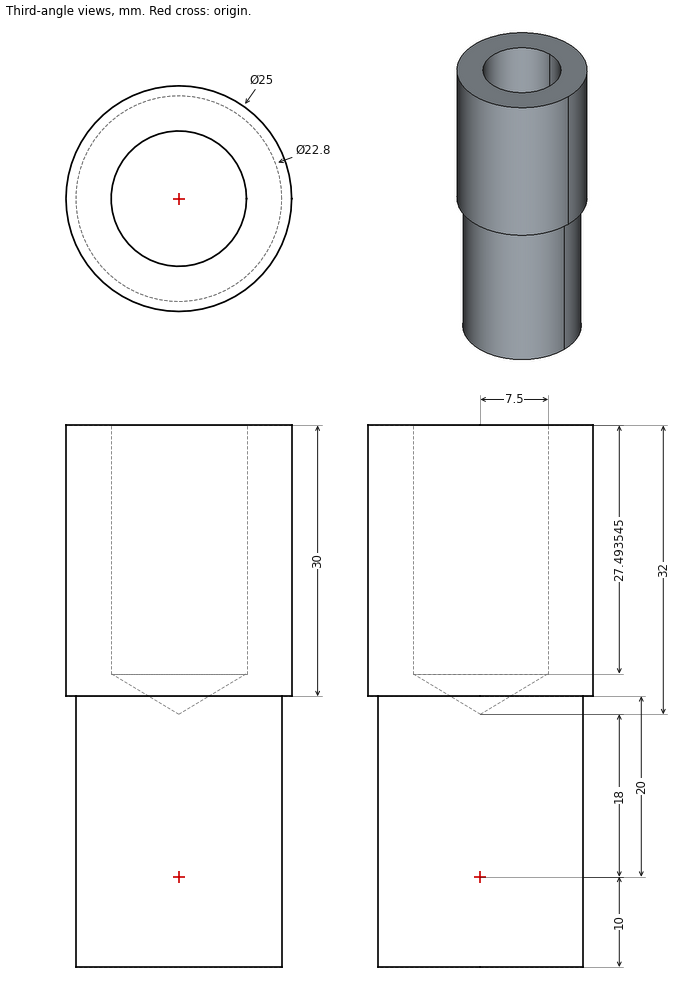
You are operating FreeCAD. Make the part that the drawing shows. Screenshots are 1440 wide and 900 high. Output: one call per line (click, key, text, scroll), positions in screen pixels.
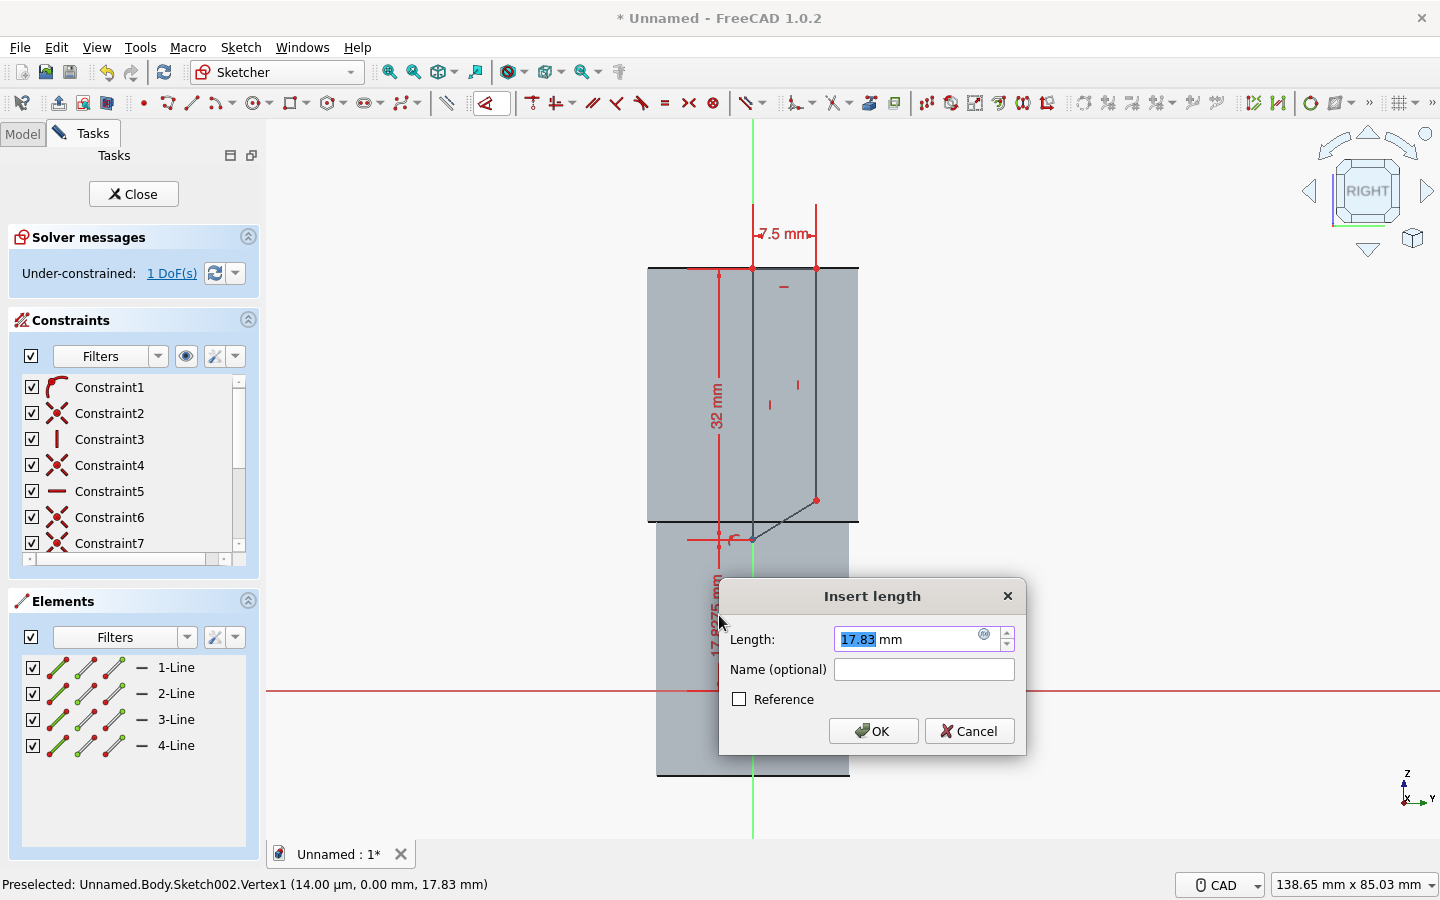
text(18)
key(Return)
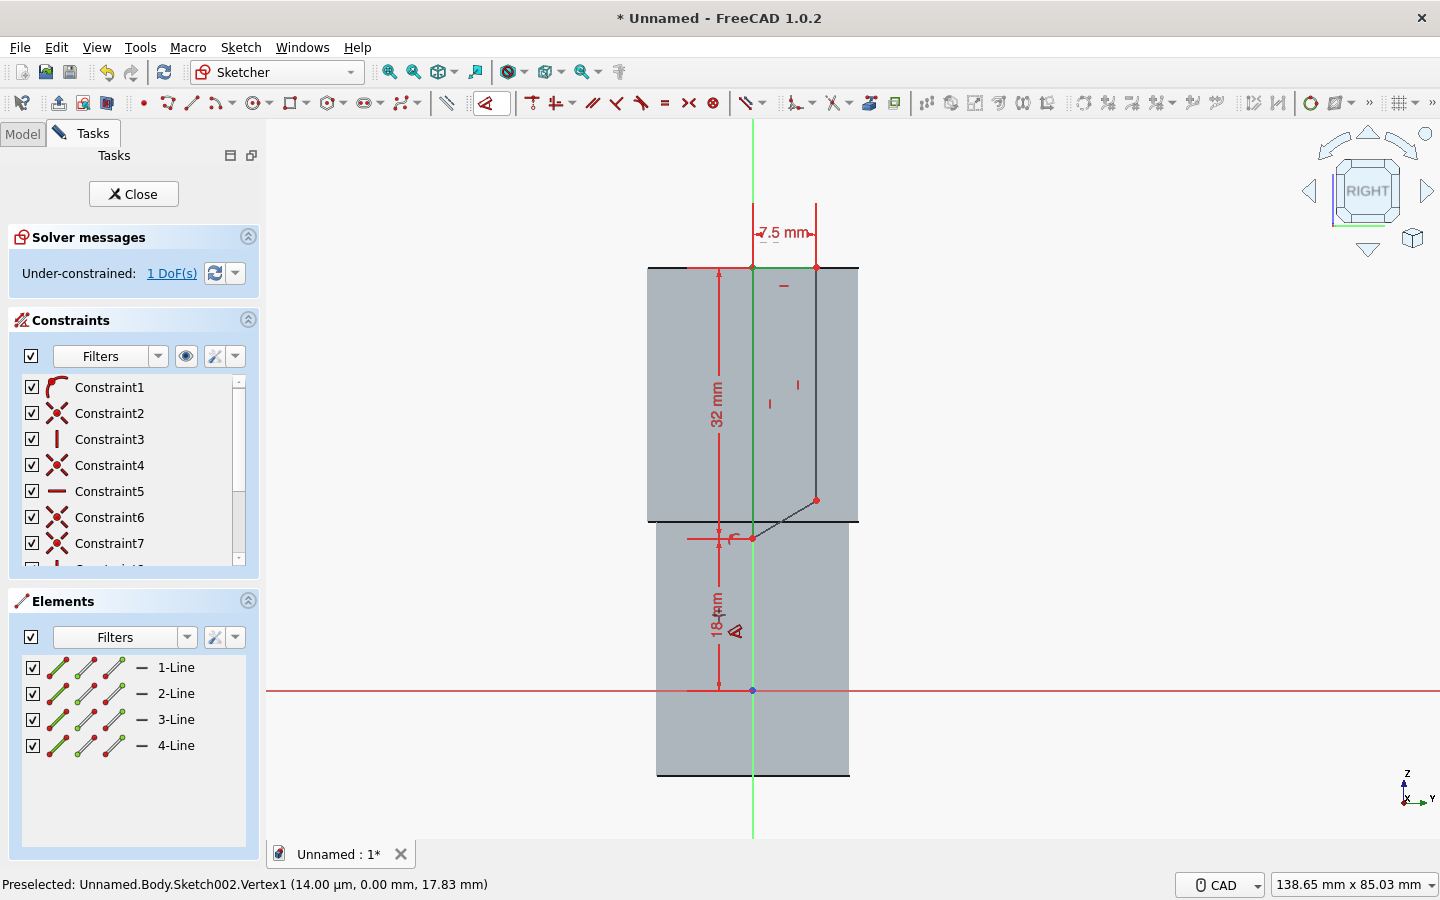
click(816, 431)
click(850, 384)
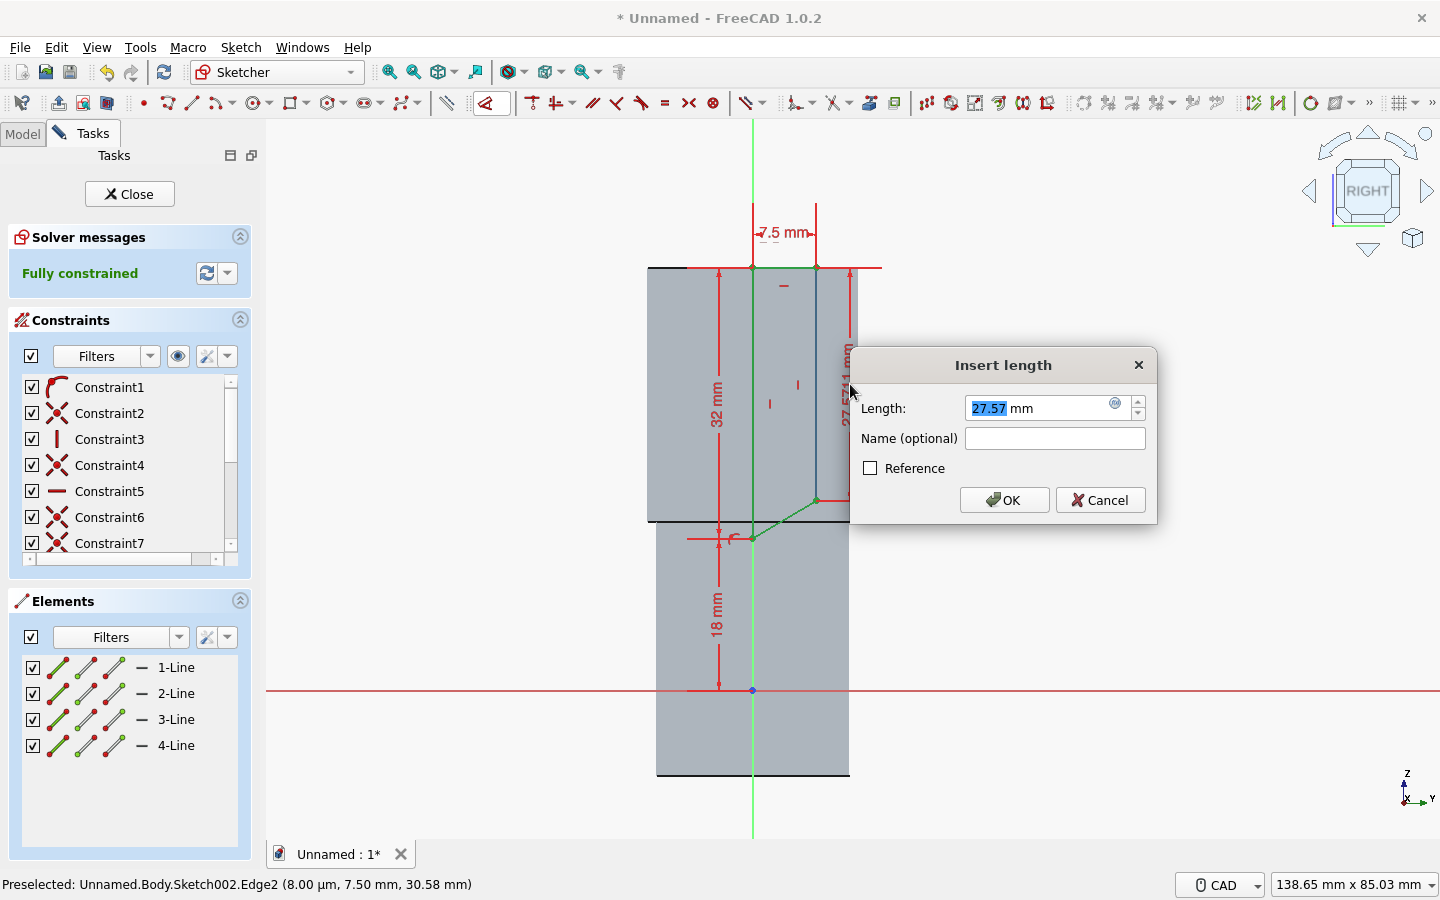
text(27.493545)
key(Return)
key(Escape)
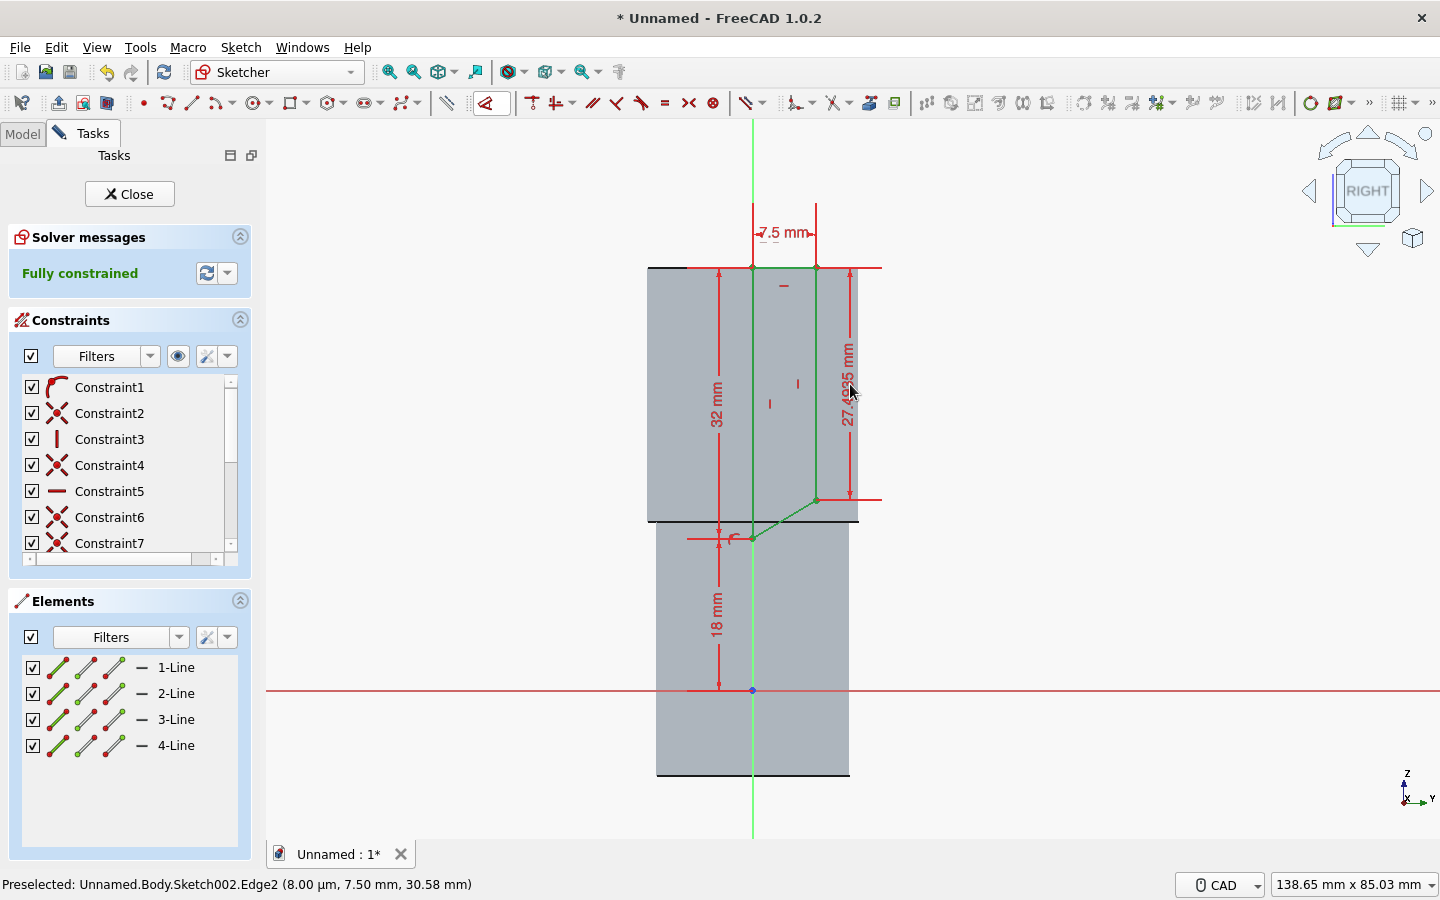
click(130, 194)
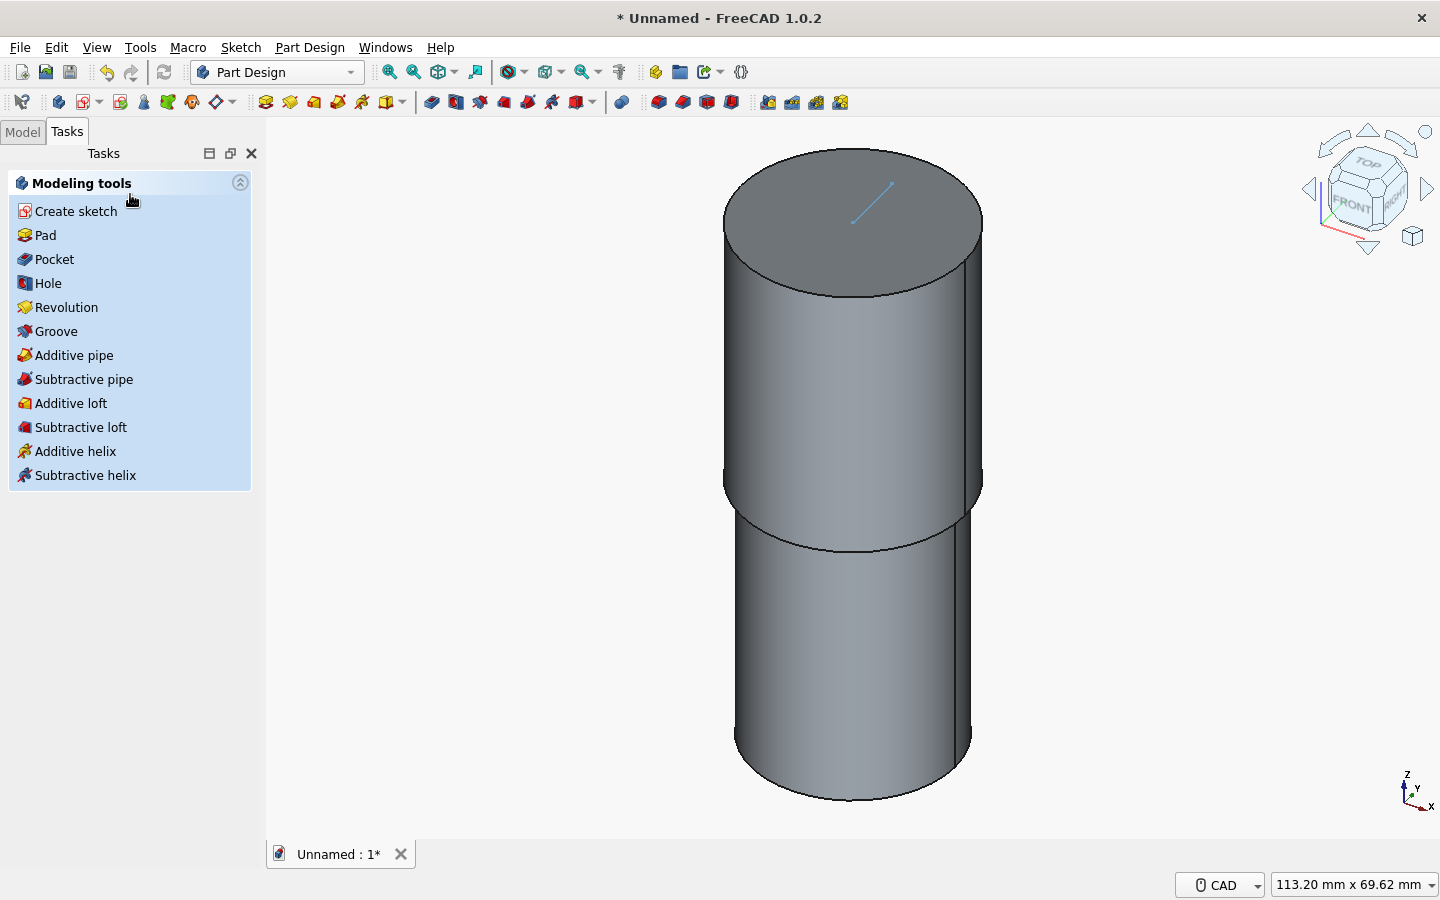
click(480, 102)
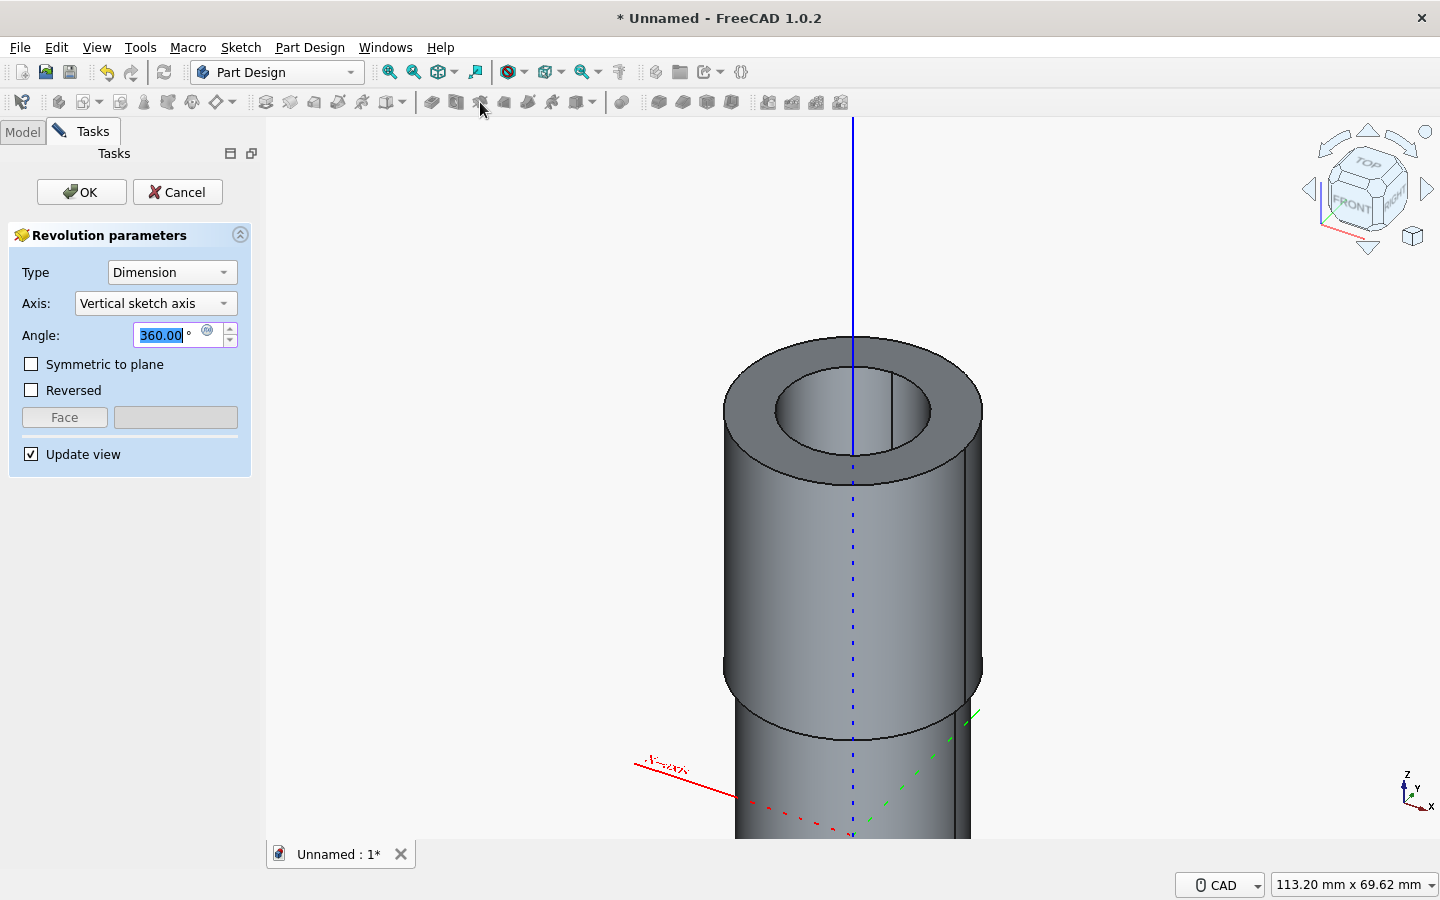
click(82, 192)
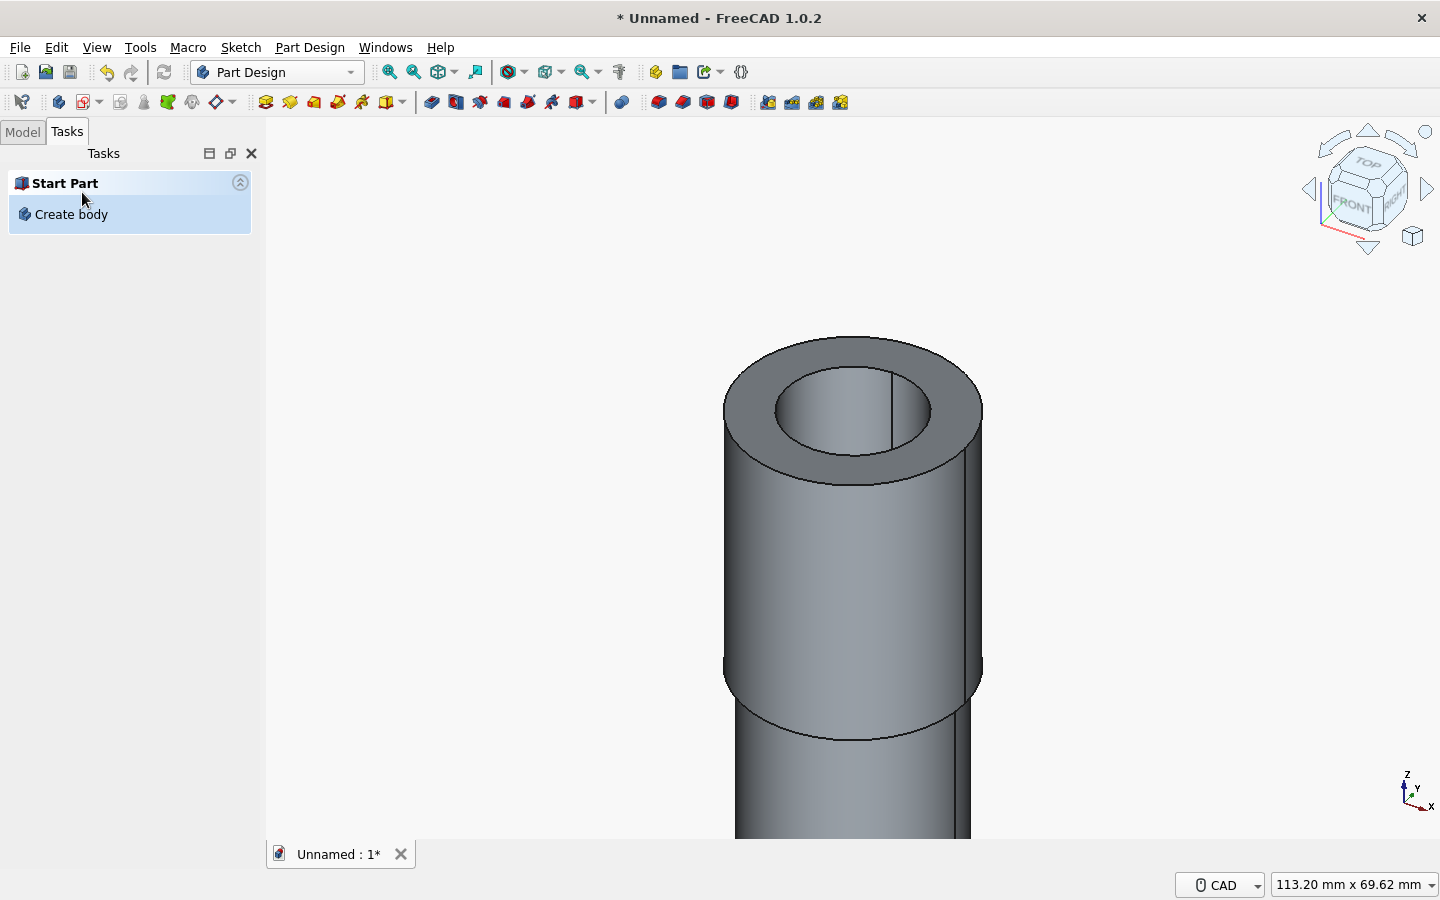
key(0)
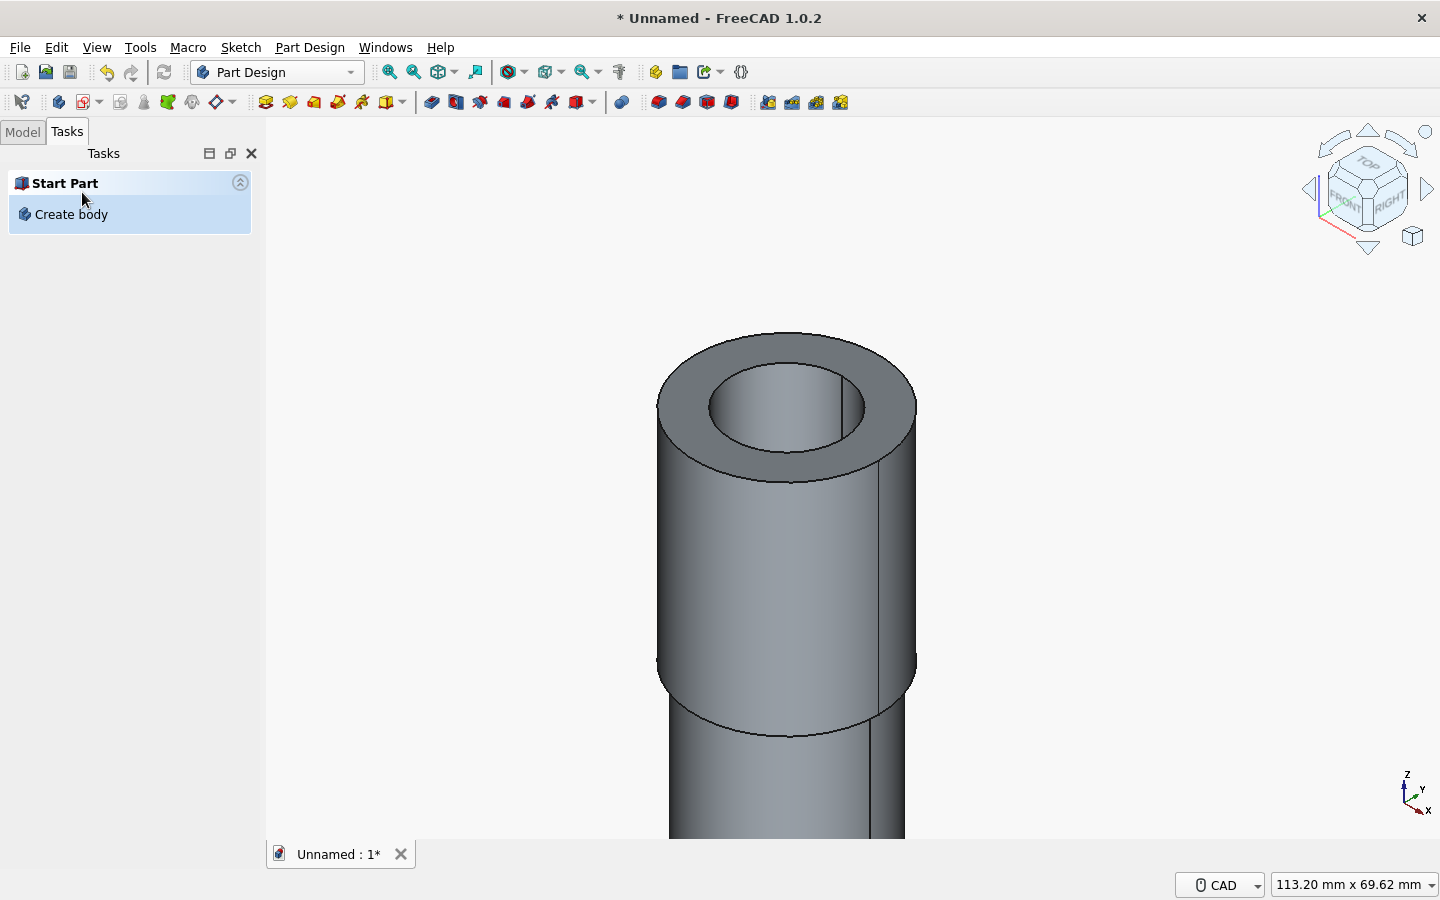
click(390, 72)